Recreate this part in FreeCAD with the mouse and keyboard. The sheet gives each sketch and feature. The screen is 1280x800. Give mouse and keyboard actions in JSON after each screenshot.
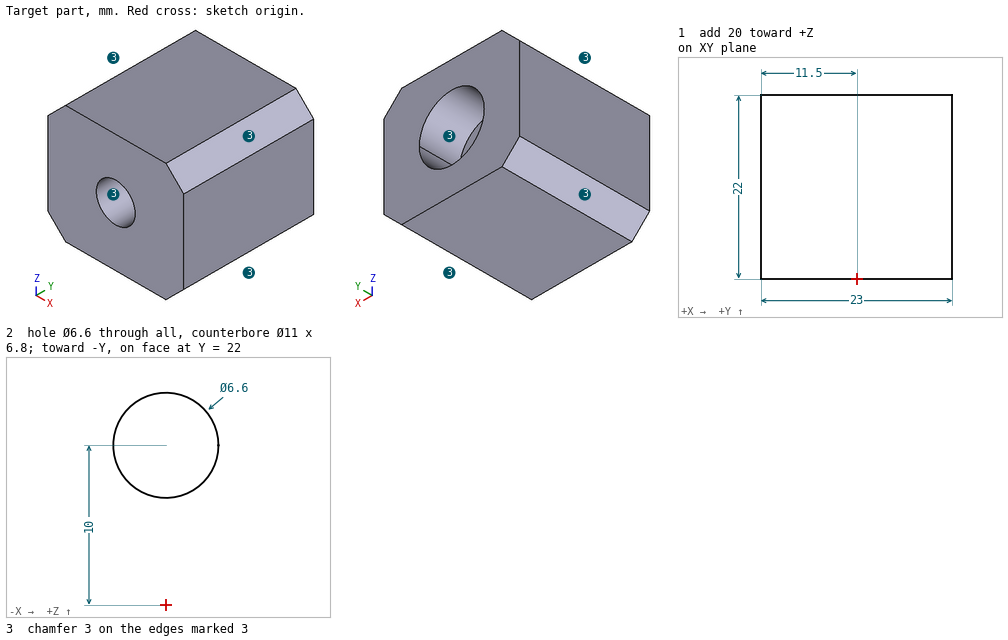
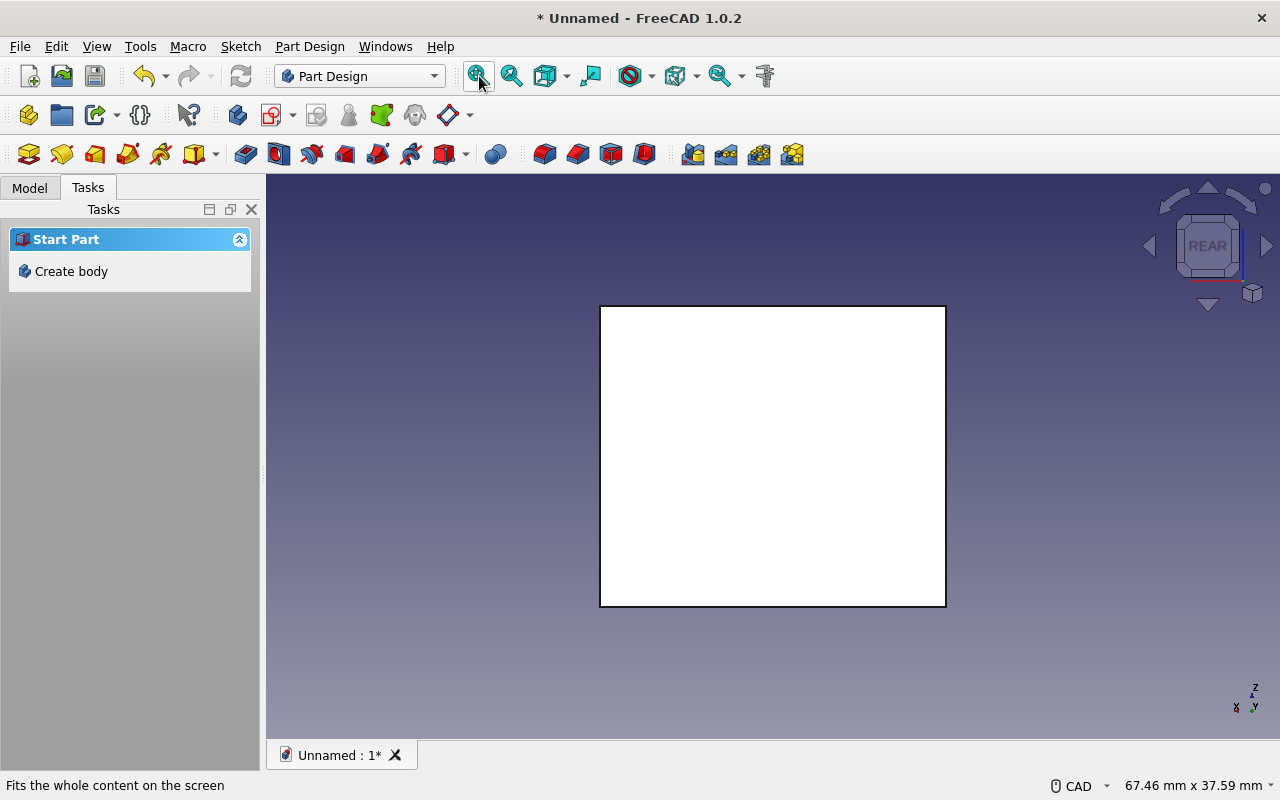
{"action": "left_click", "coordinate": [773, 455]}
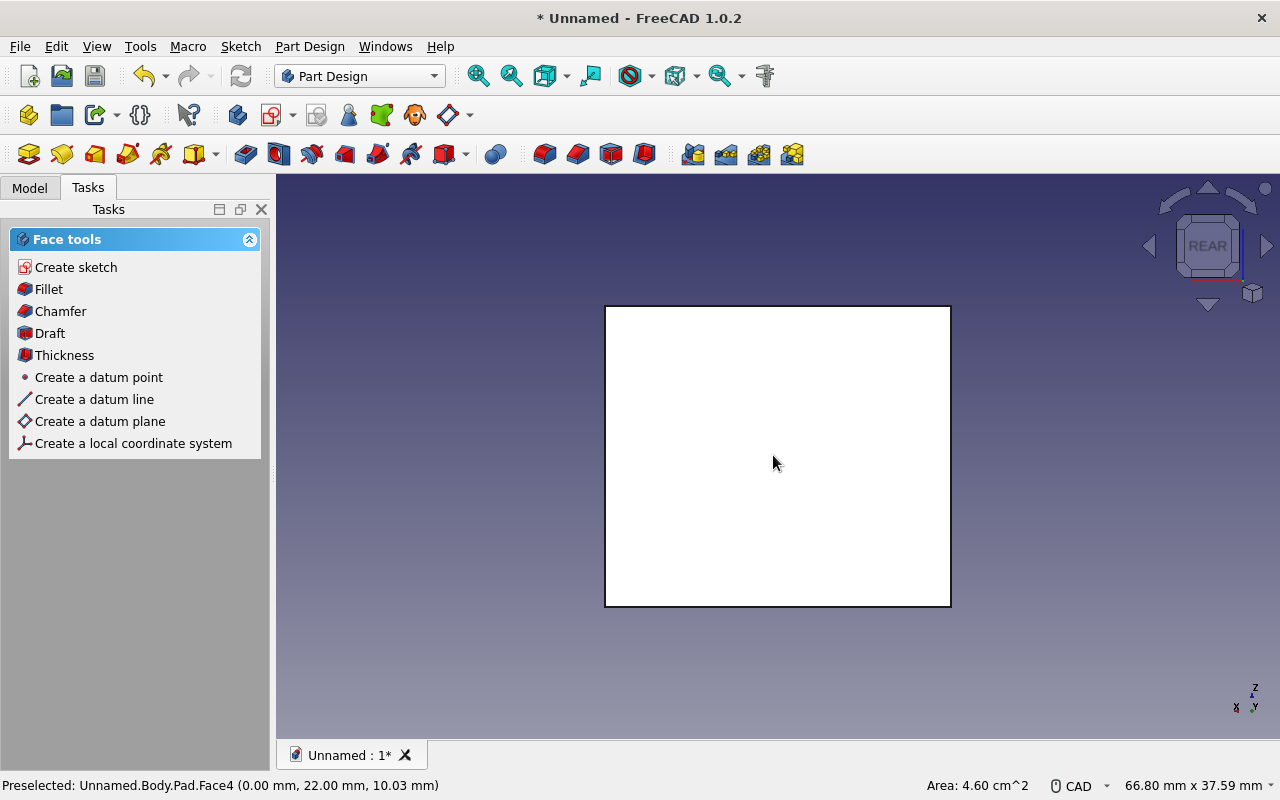
{"action": "left_click", "coordinate": [270, 116]}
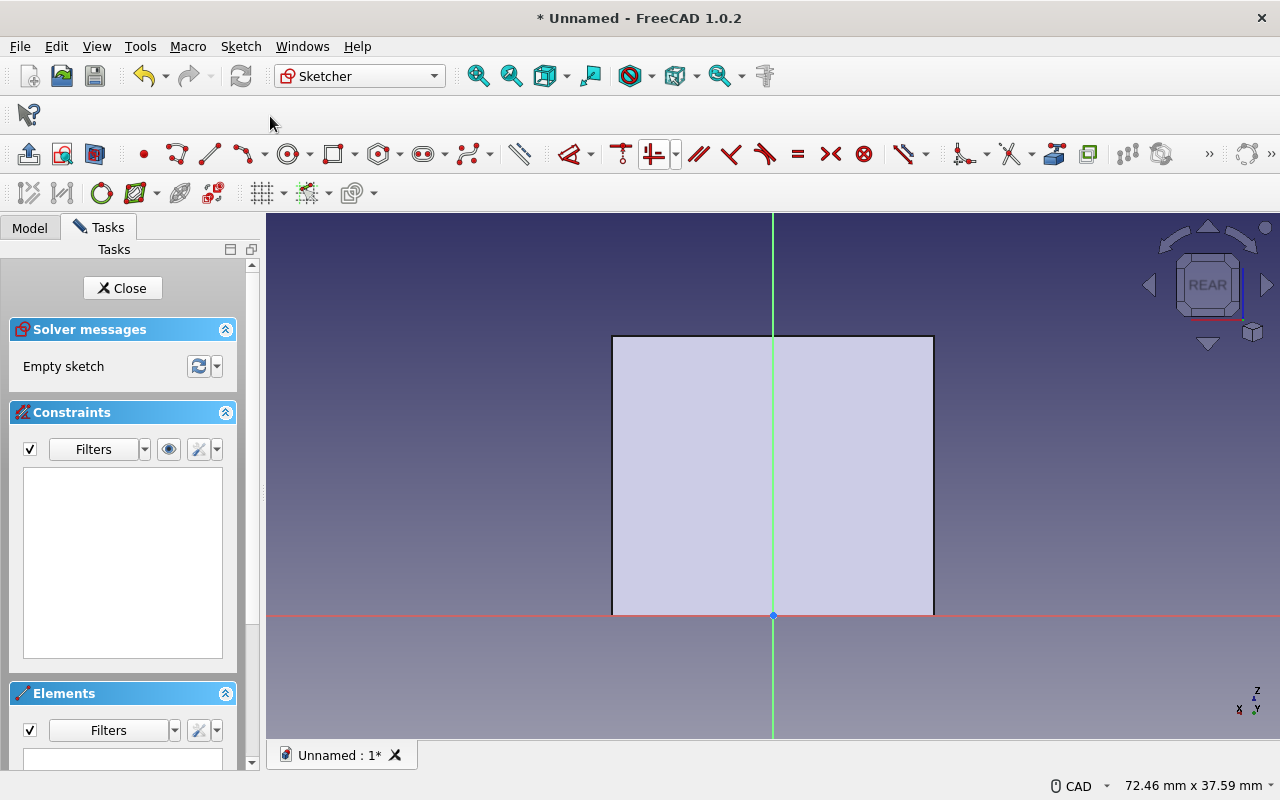
{"action": "scroll", "coordinate": [856, 580], "scroll_direction": "up", "scroll_amount": 3}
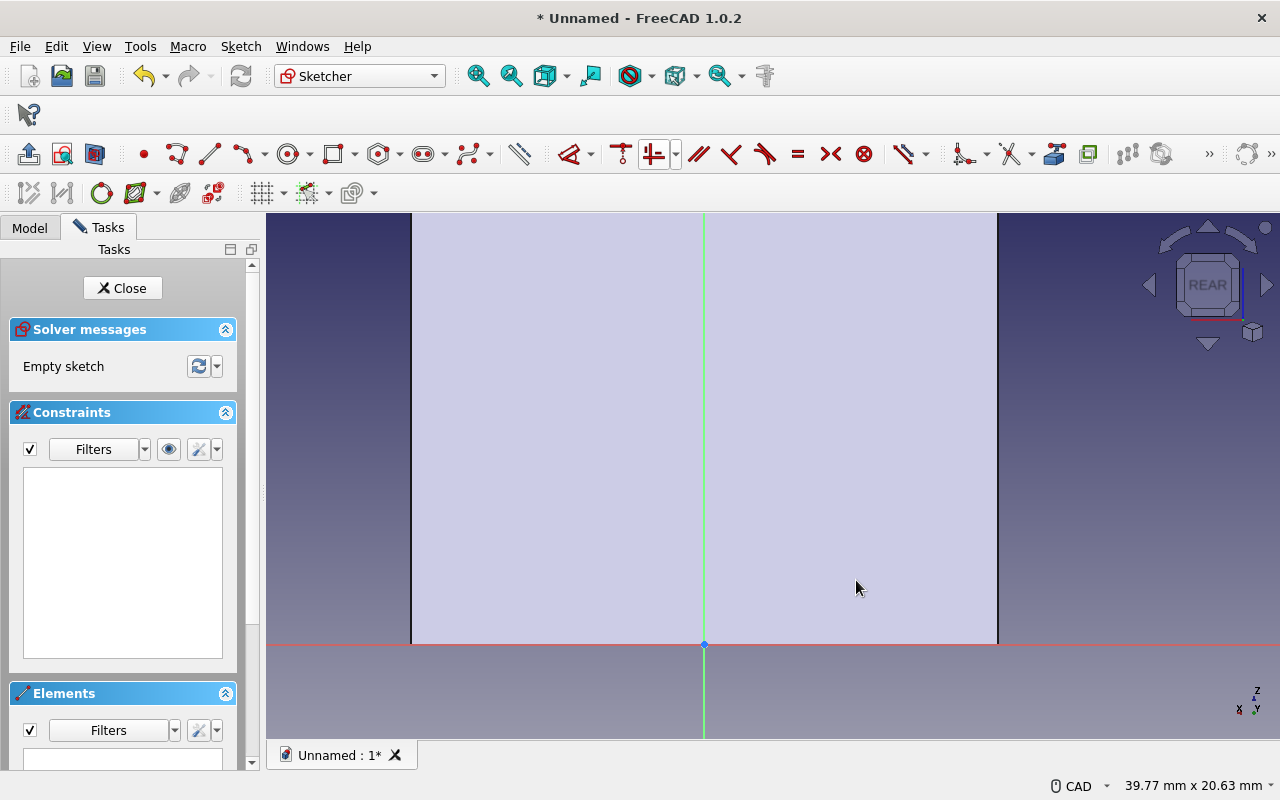
{"action": "left_click", "coordinate": [288, 154]}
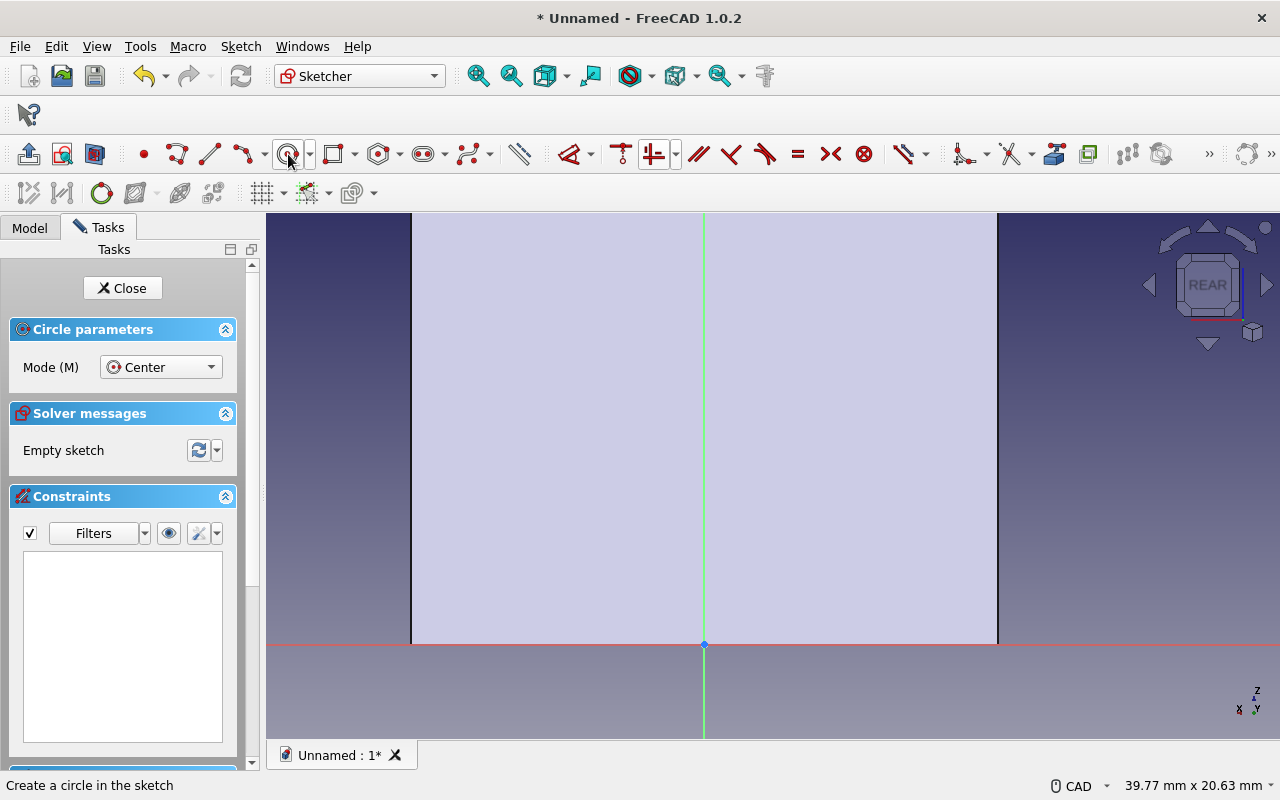
{"action": "left_click", "coordinate": [704, 390]}
{"action": "mouse_move", "coordinate": [764, 330]}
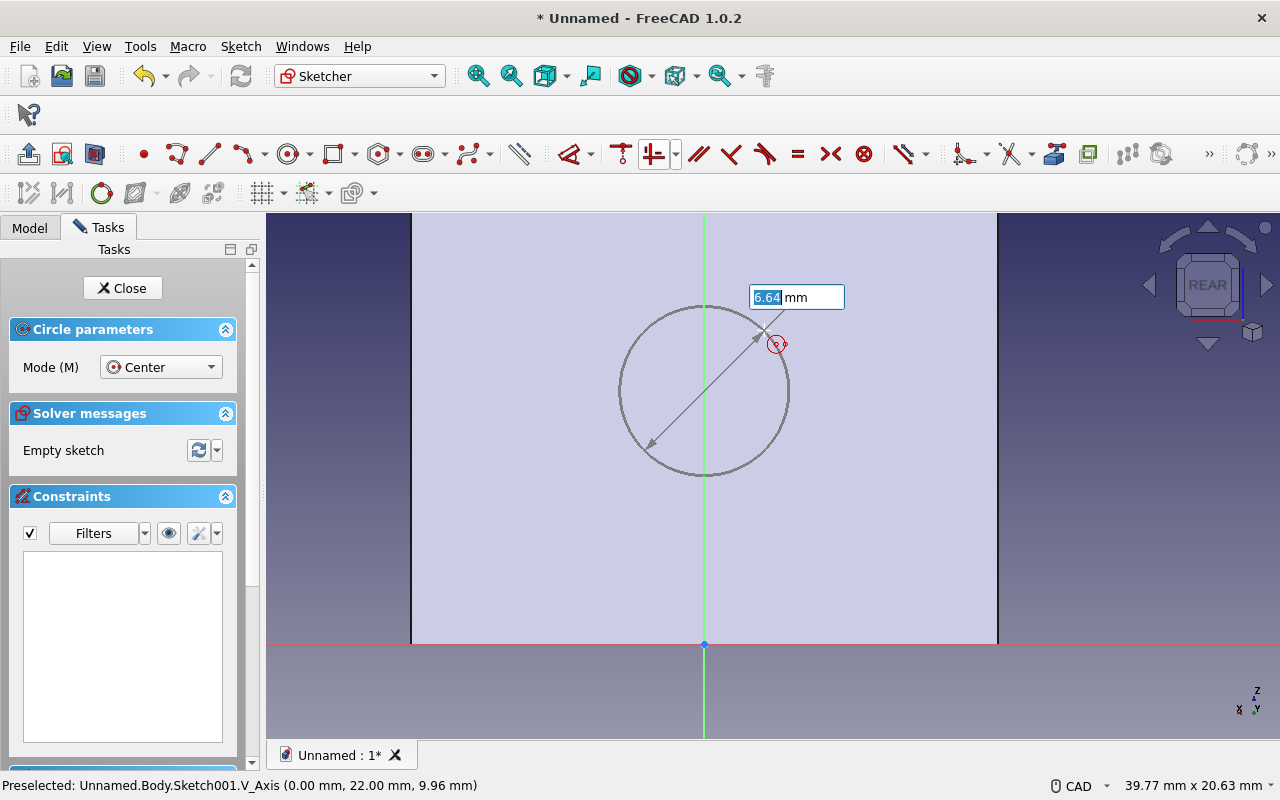
{"action": "type", "text": "6.6"}
{"action": "key", "text": "Return"}
{"action": "key", "text": "Escape"}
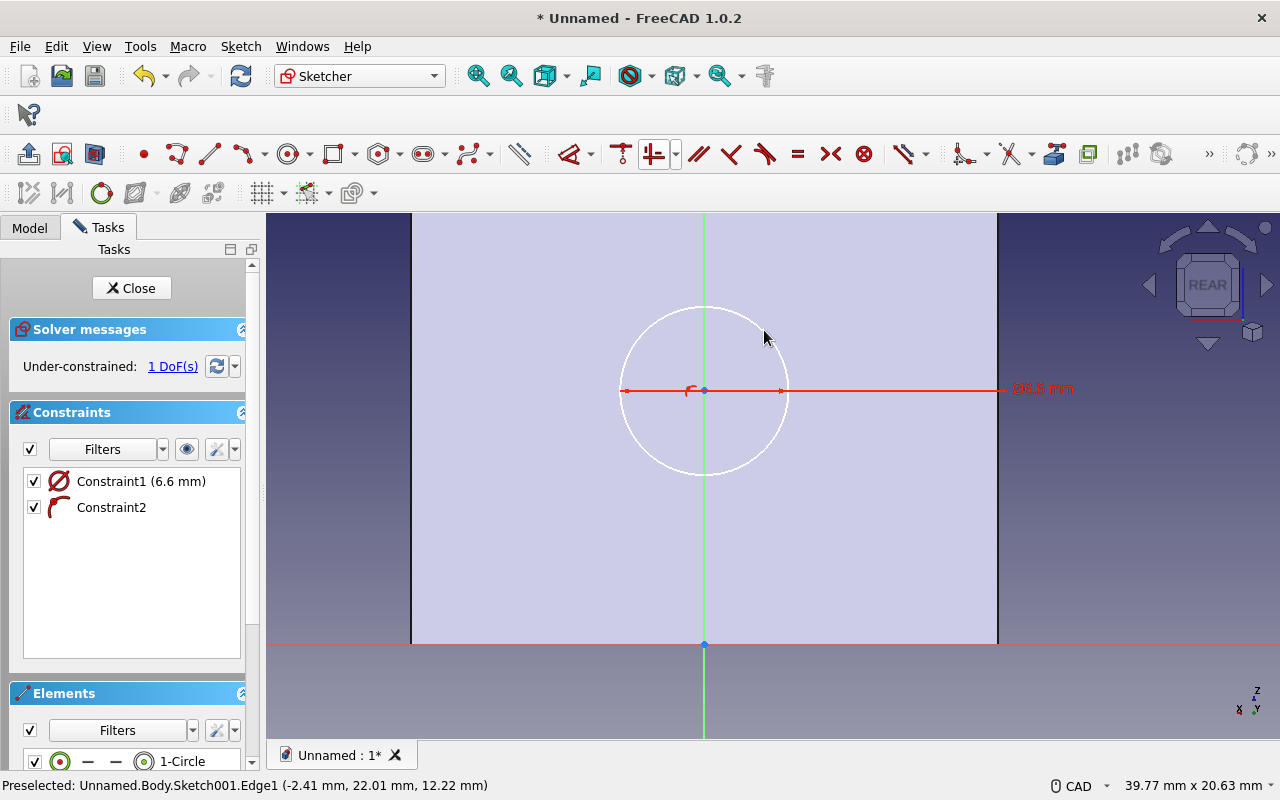
{"action": "left_click", "coordinate": [568, 154]}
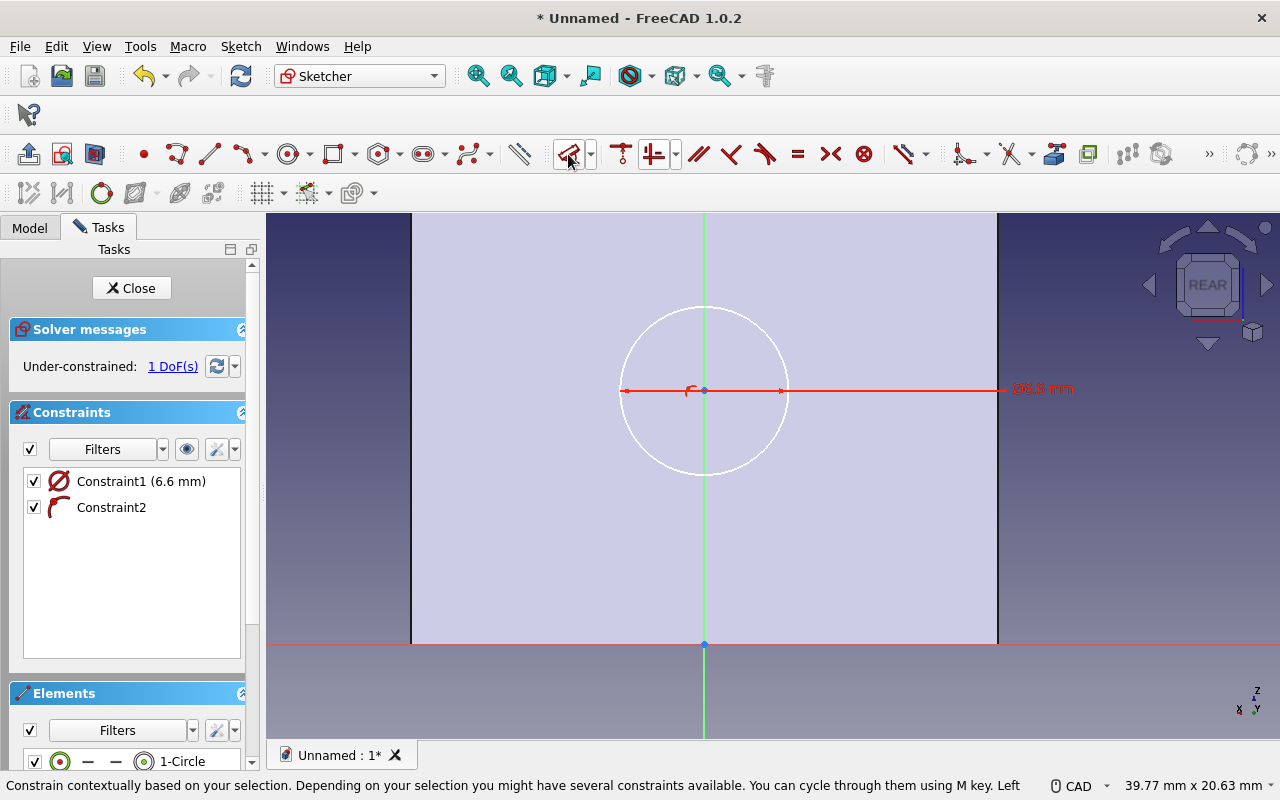
{"action": "left_click", "coordinate": [704, 391]}
{"action": "left_click", "coordinate": [738, 518]}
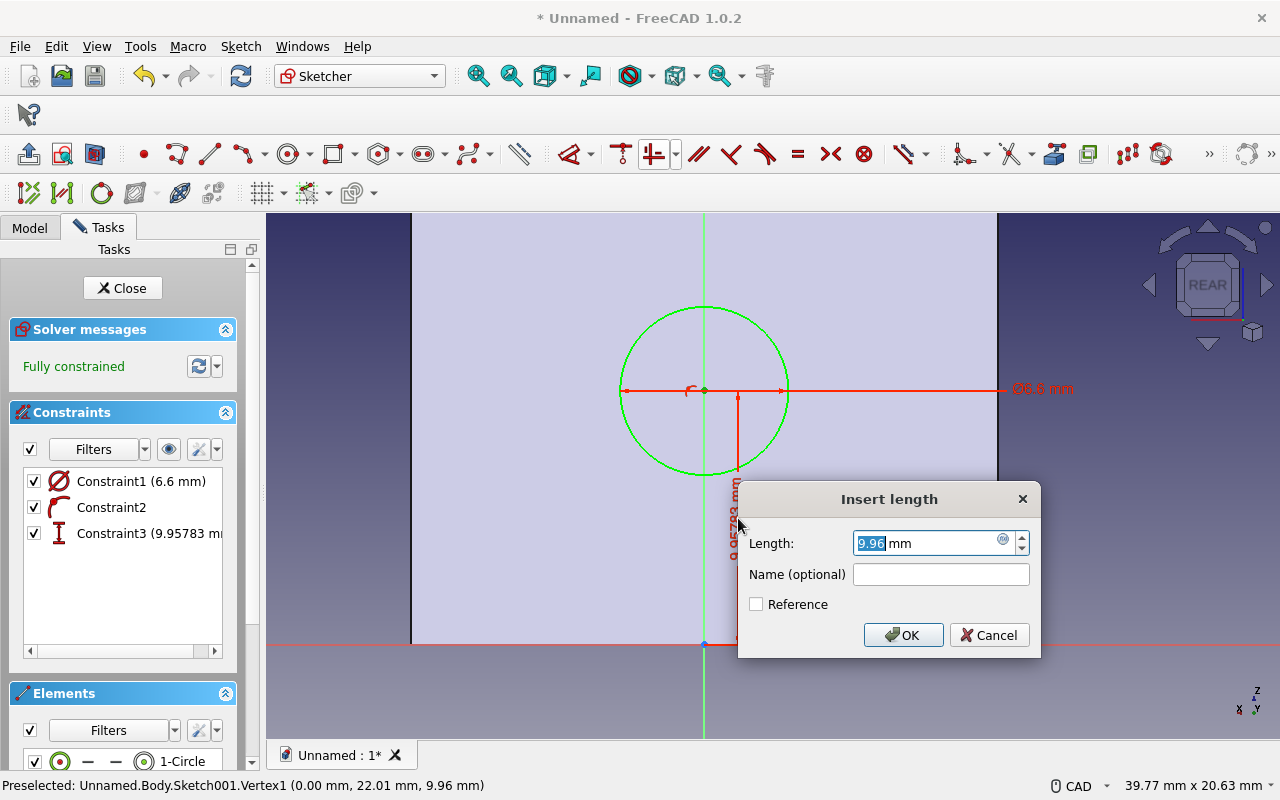
{"action": "type", "text": "10"}
{"action": "key", "text": "Return"}
{"action": "key", "text": "Escape"}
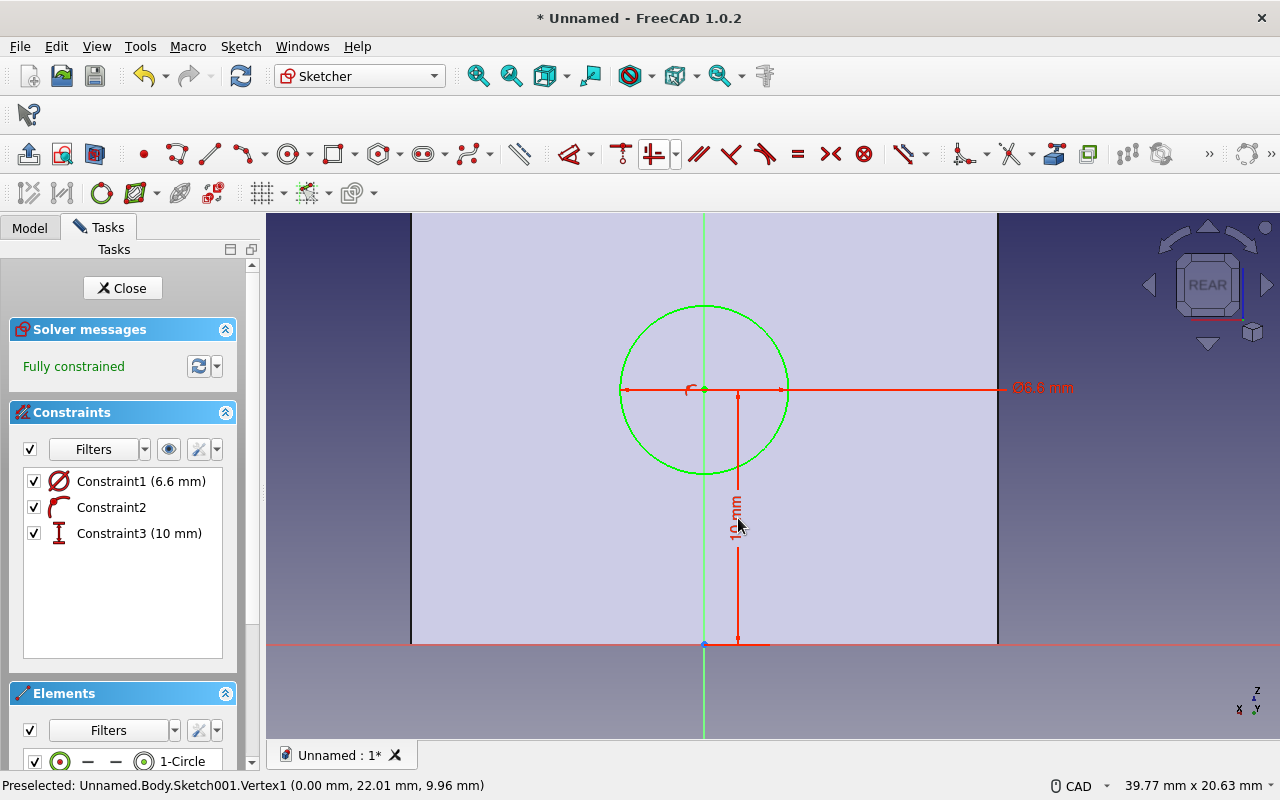
{"action": "left_click", "coordinate": [123, 288]}